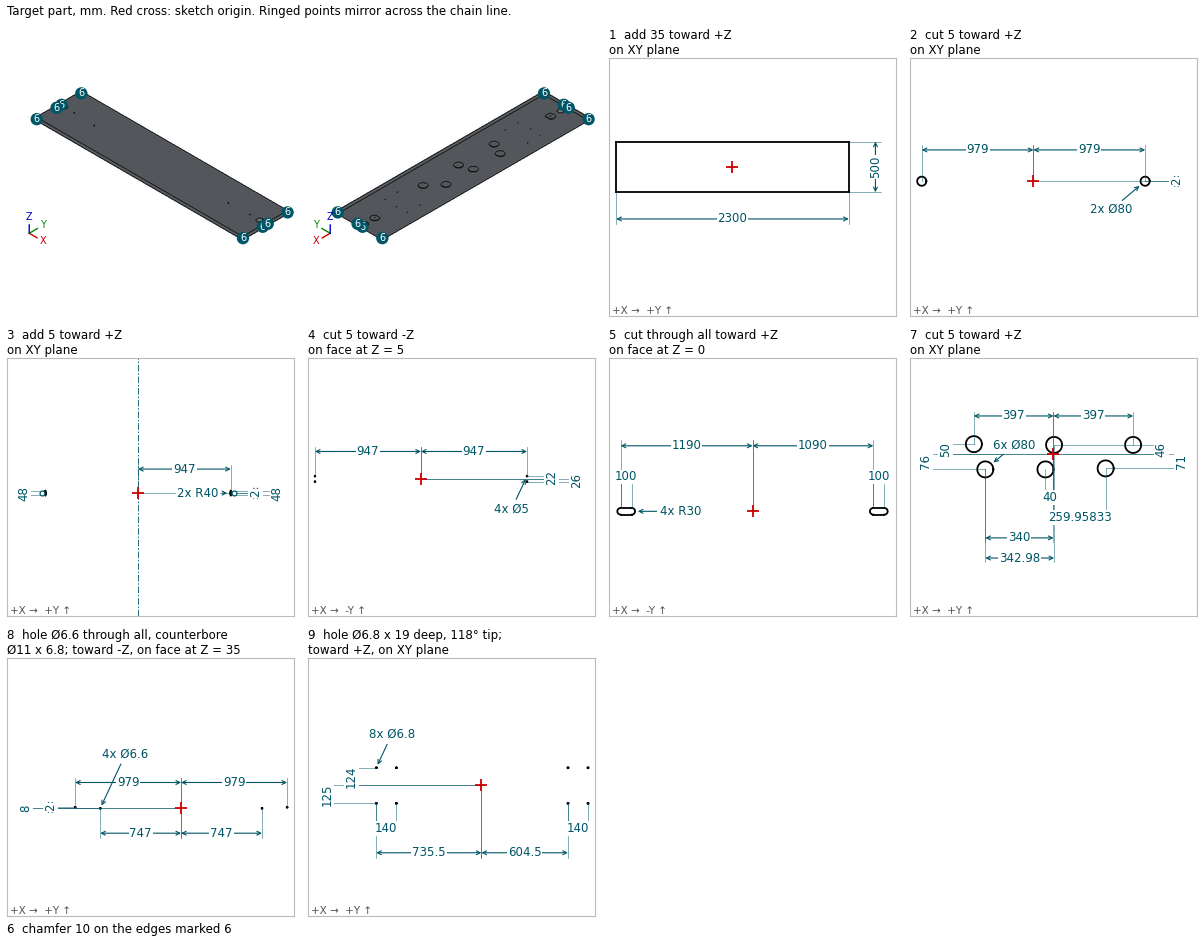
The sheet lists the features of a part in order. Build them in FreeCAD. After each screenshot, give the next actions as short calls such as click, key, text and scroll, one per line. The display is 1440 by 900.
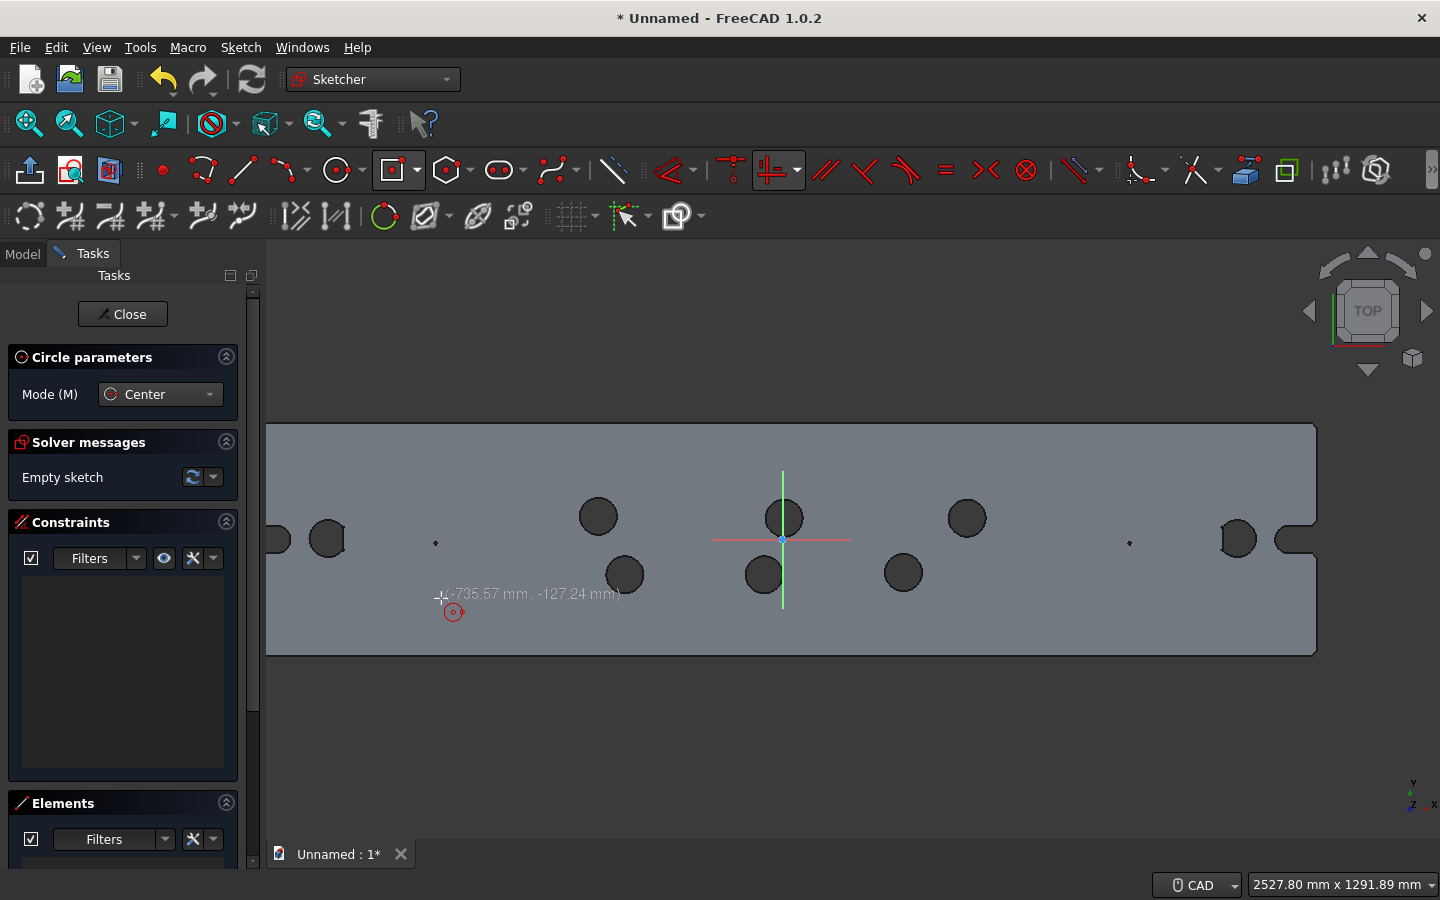
click(441, 598)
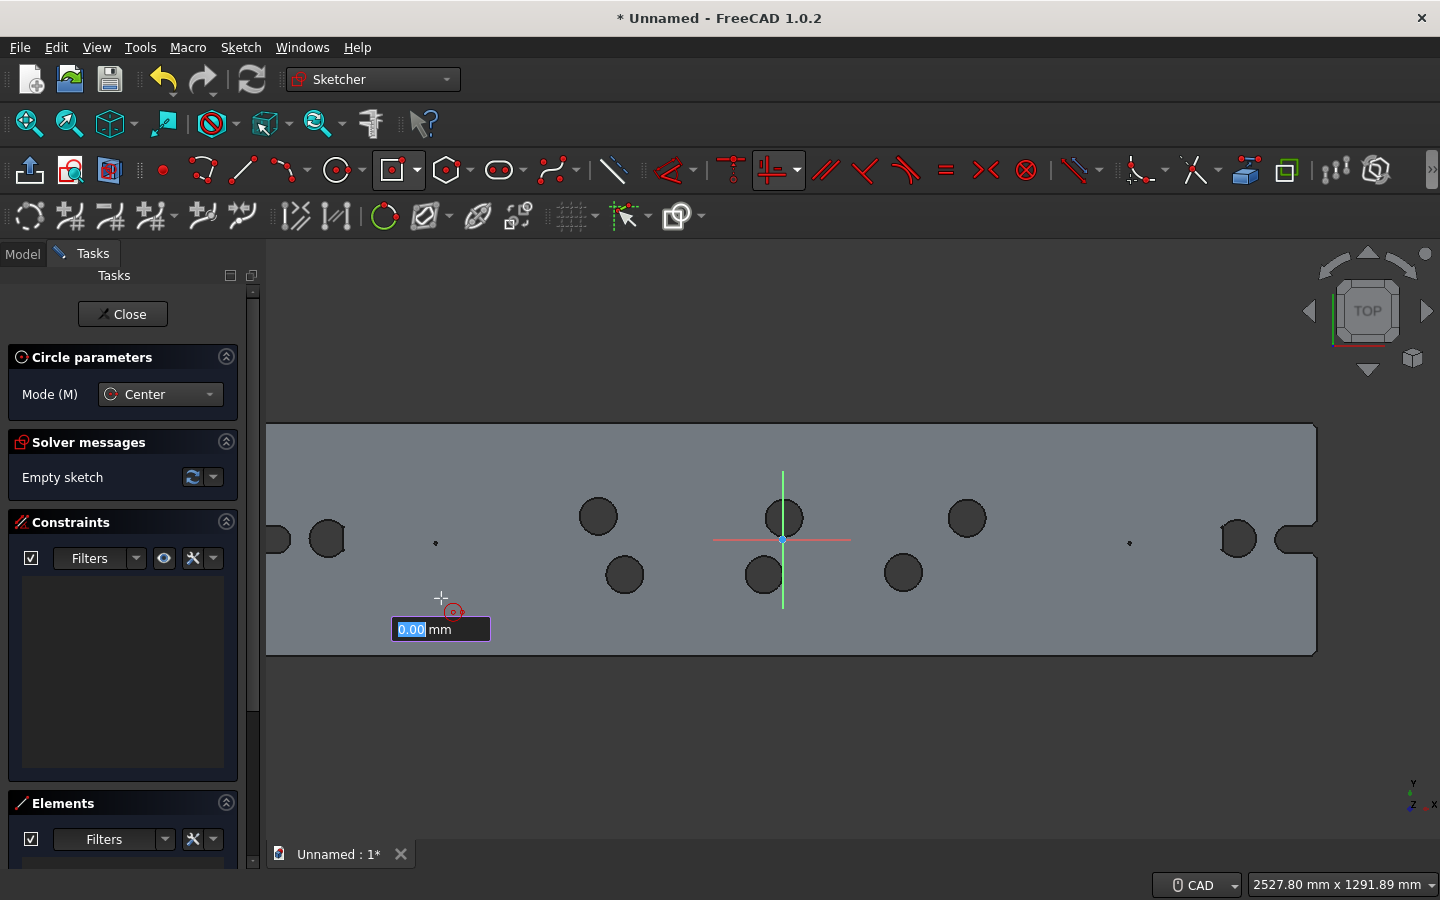
scroll(442, 596, up, 12)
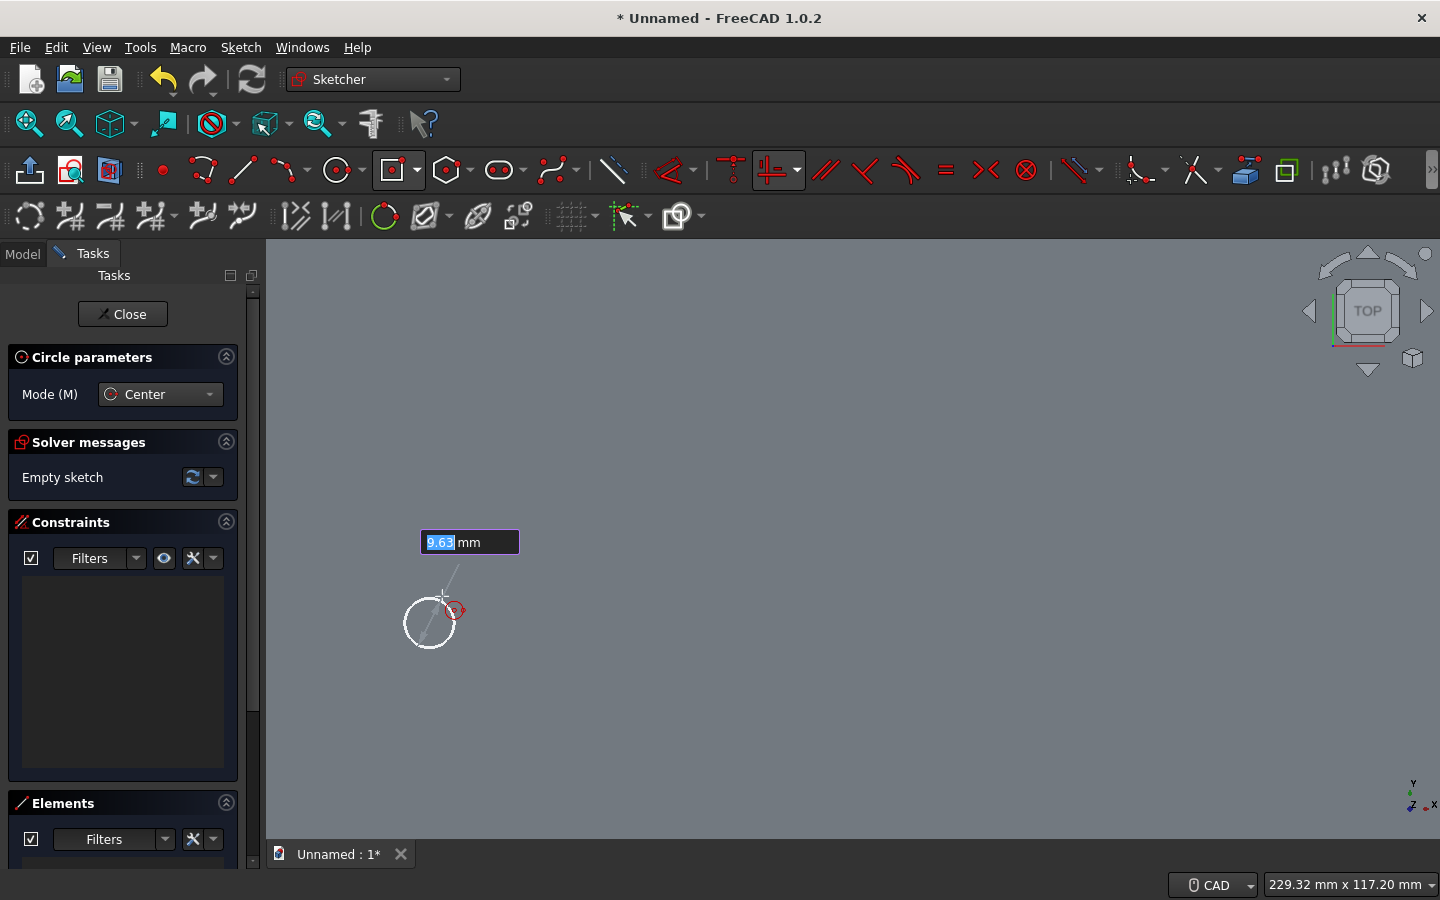
click(444, 595)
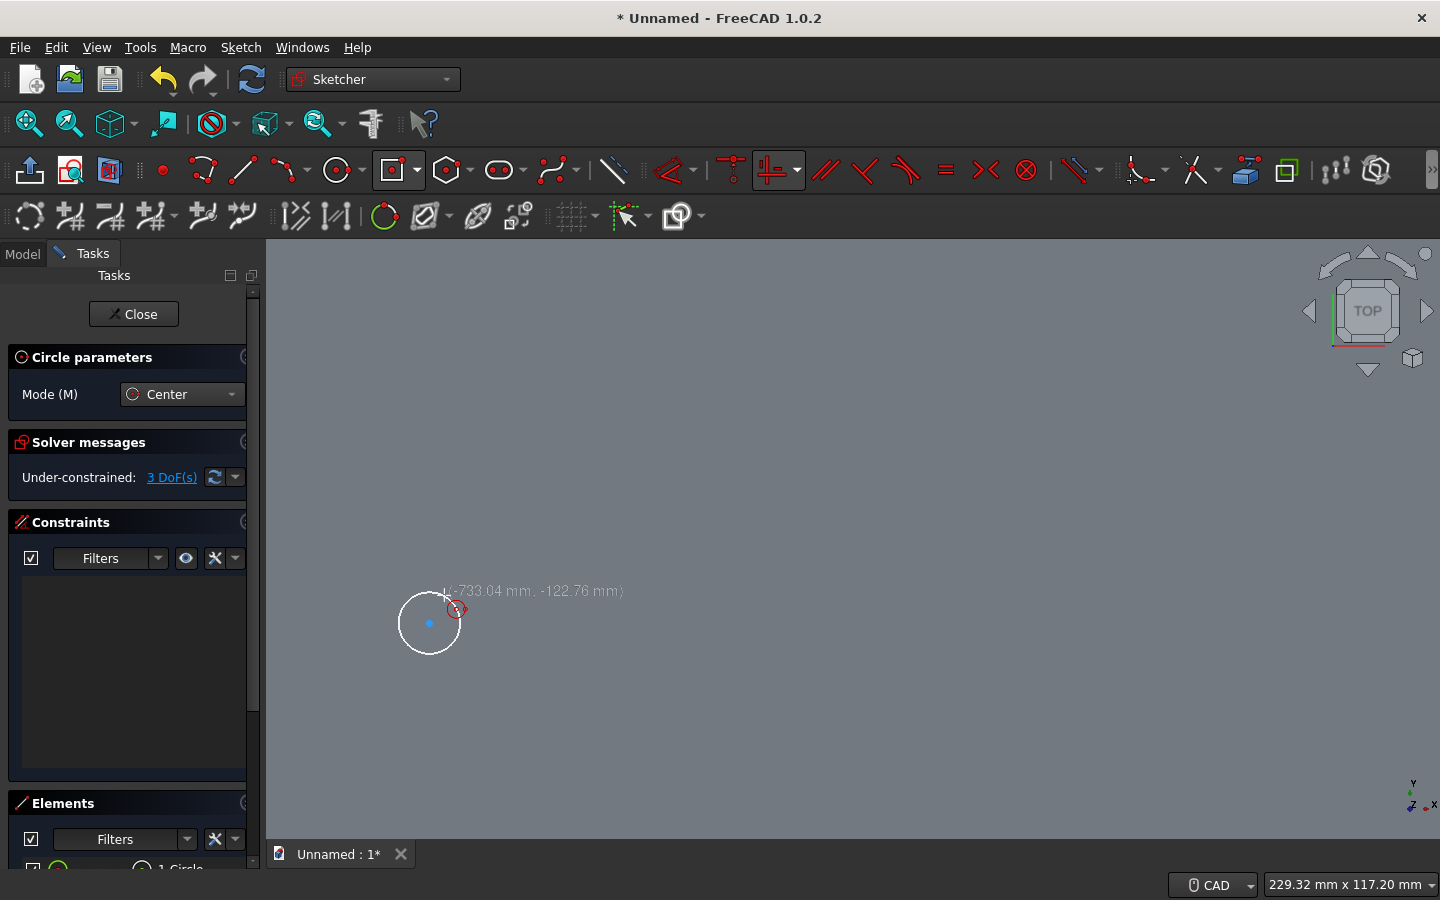
scroll(1148, 607, up, 2)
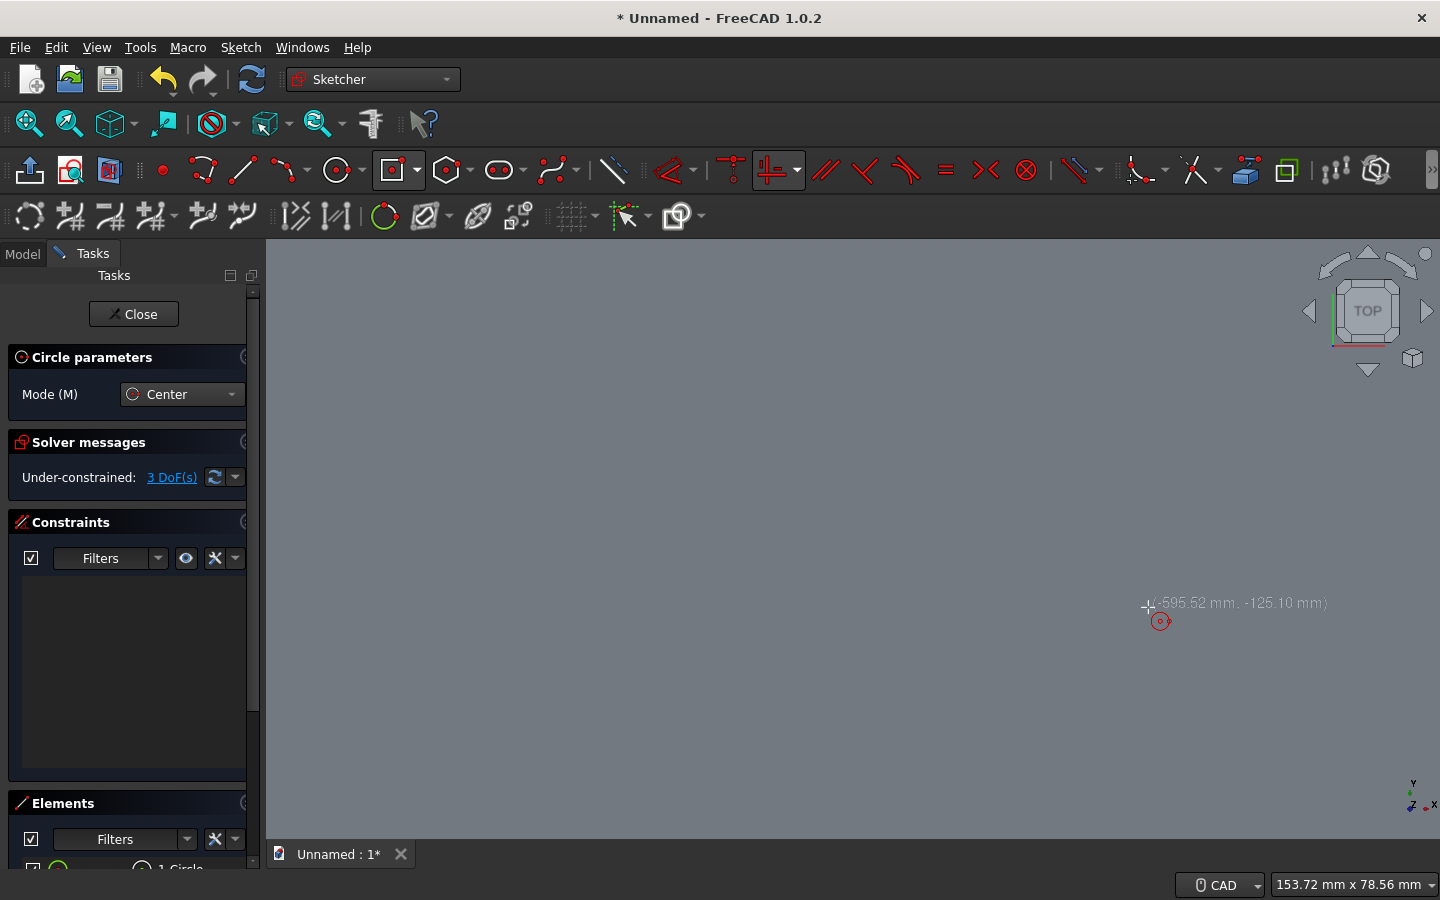
scroll(464, 596, down, 14)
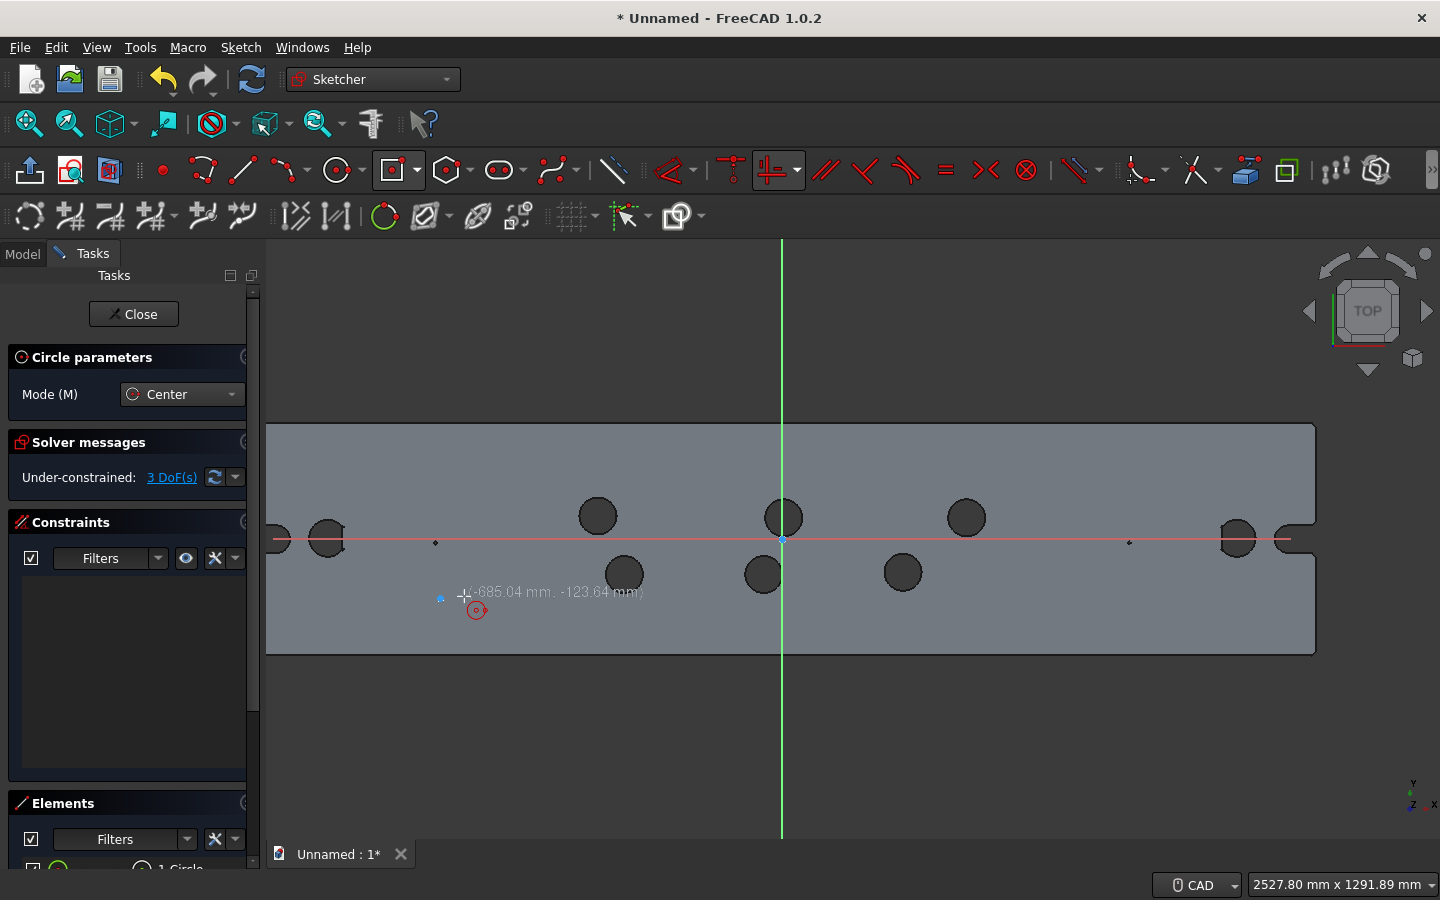
click(506, 597)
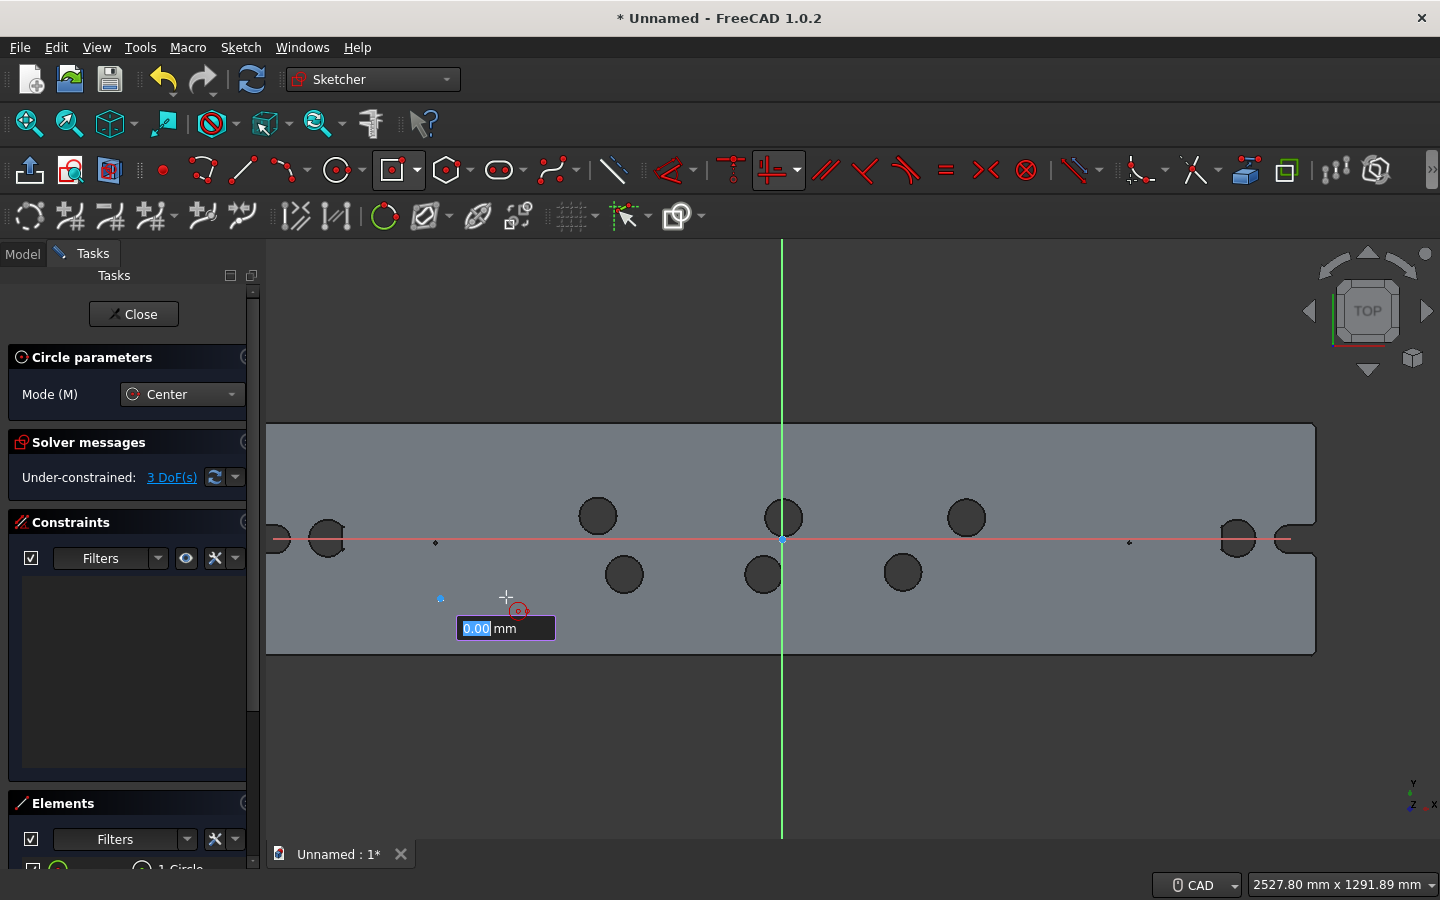
scroll(507, 596, up, 12)